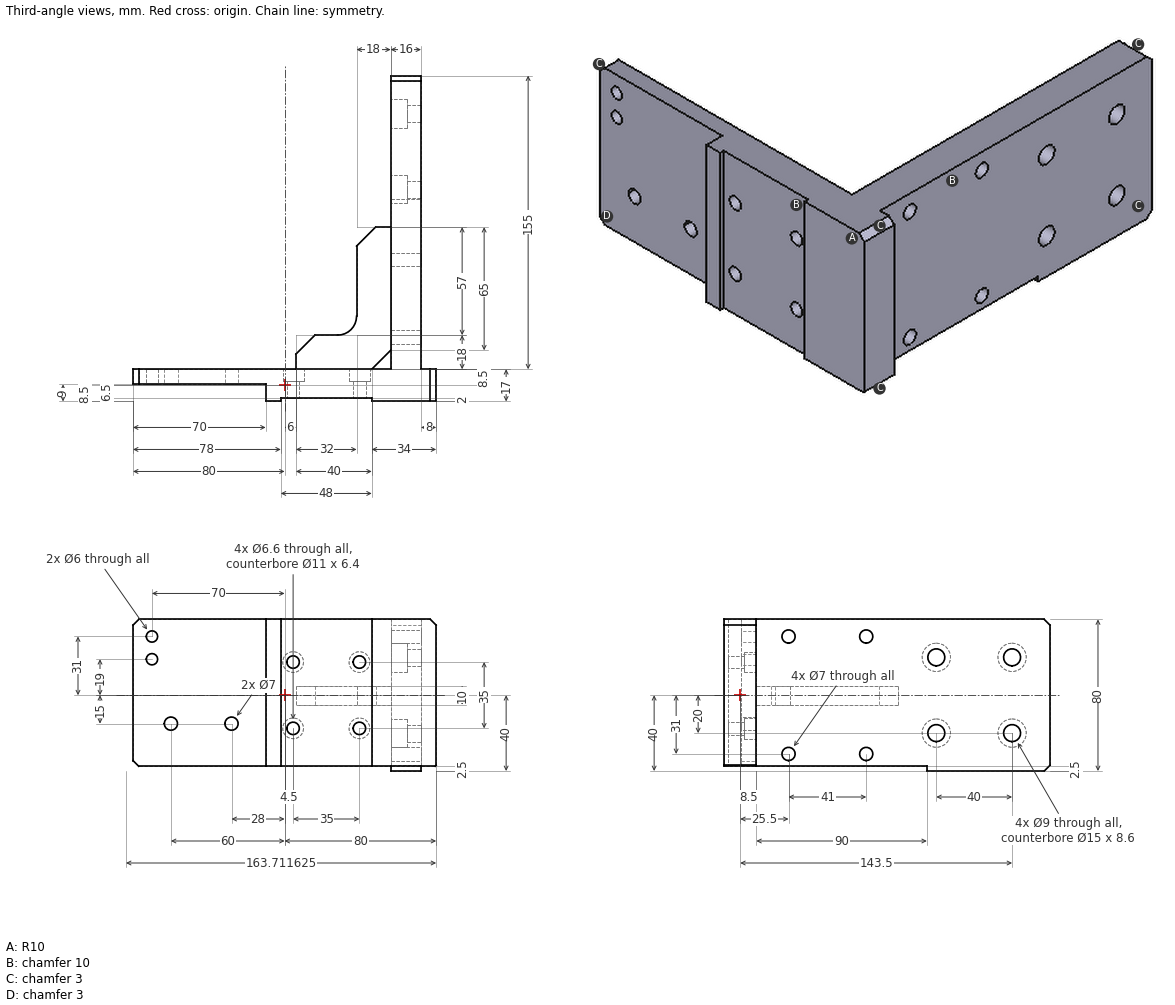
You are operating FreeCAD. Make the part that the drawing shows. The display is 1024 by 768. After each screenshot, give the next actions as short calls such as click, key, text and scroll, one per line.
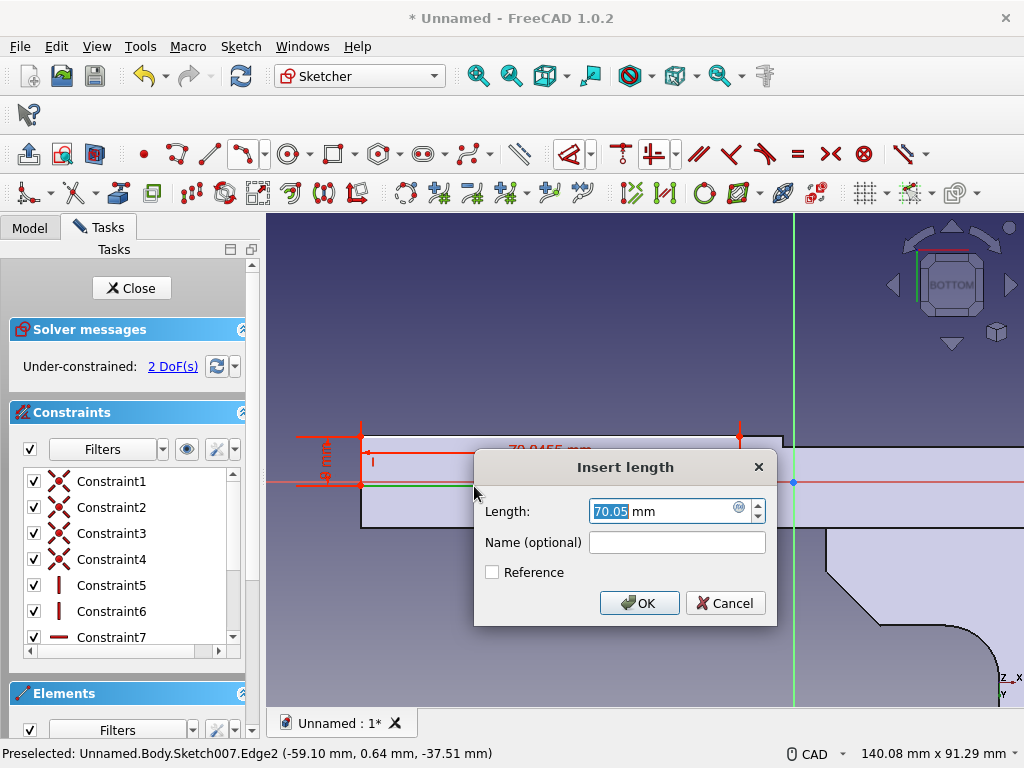
text(70)
key(Return)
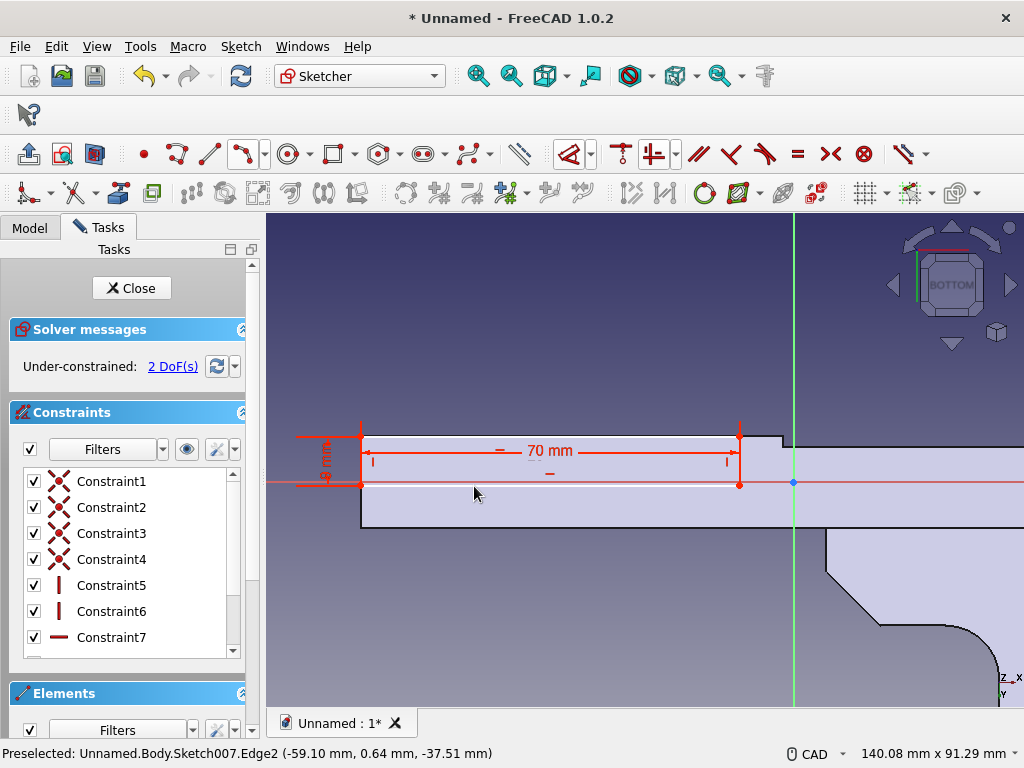
click(361, 437)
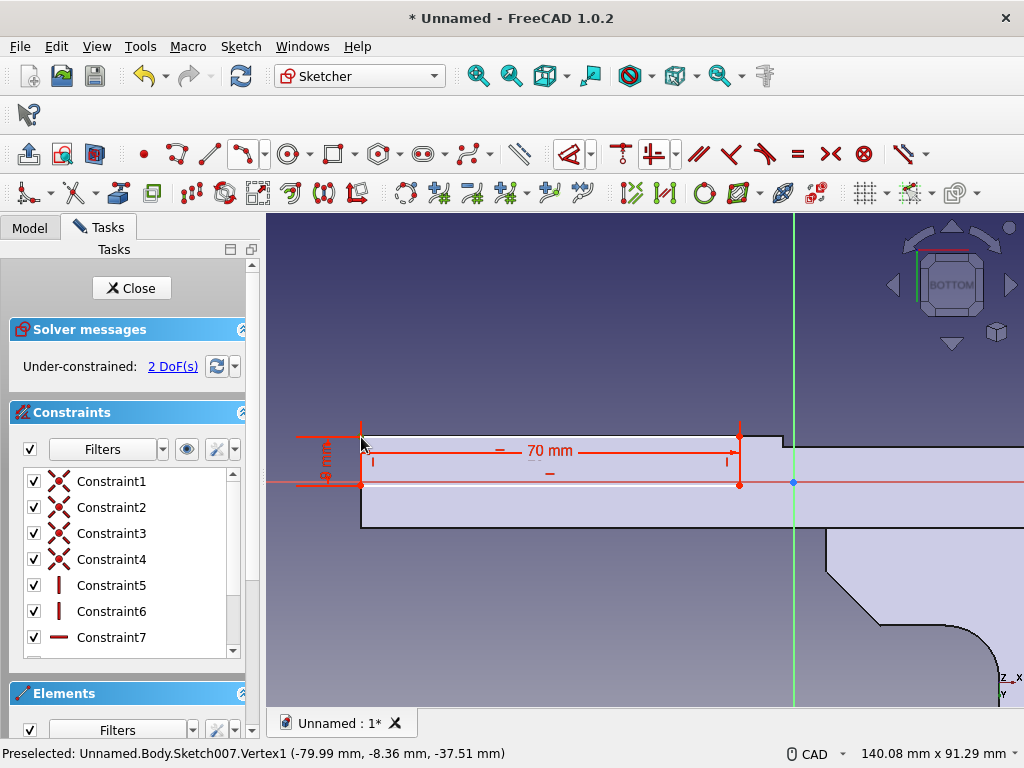
click(590, 154)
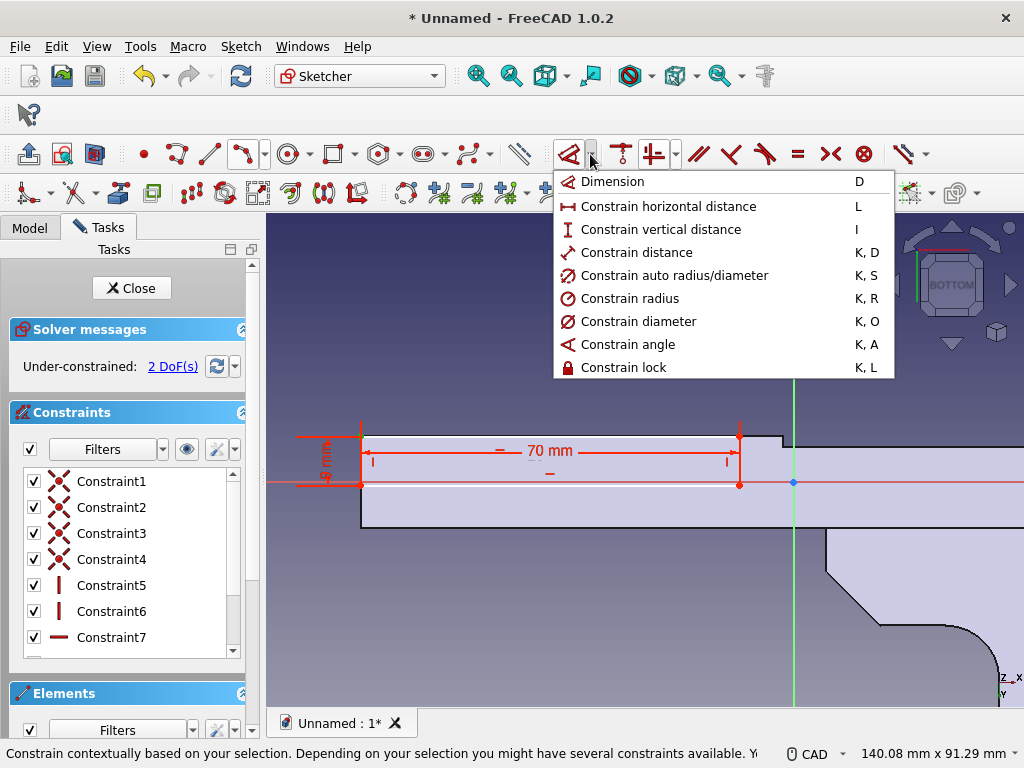
click(724, 206)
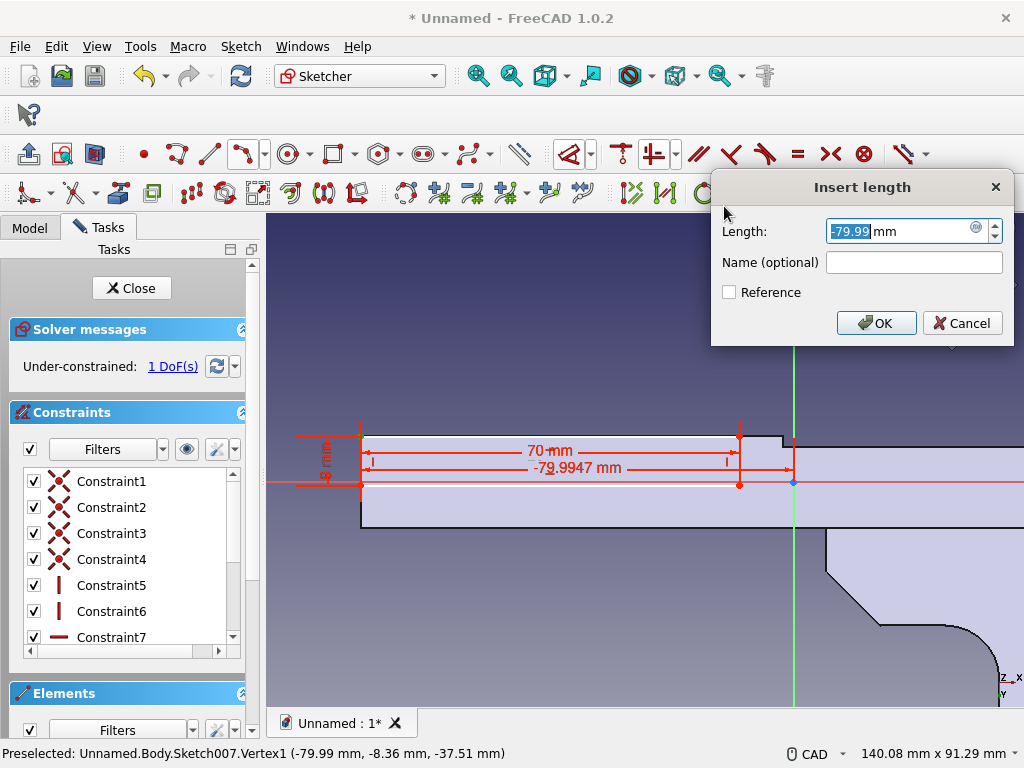
text(-80)
key(Return)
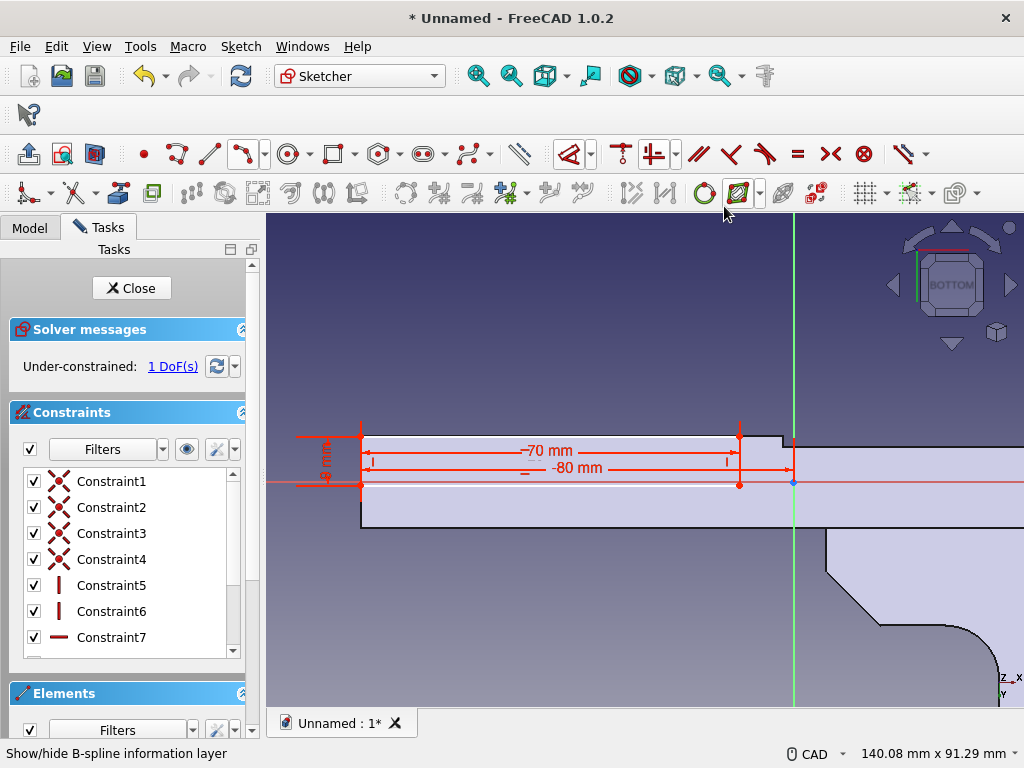
click(361, 437)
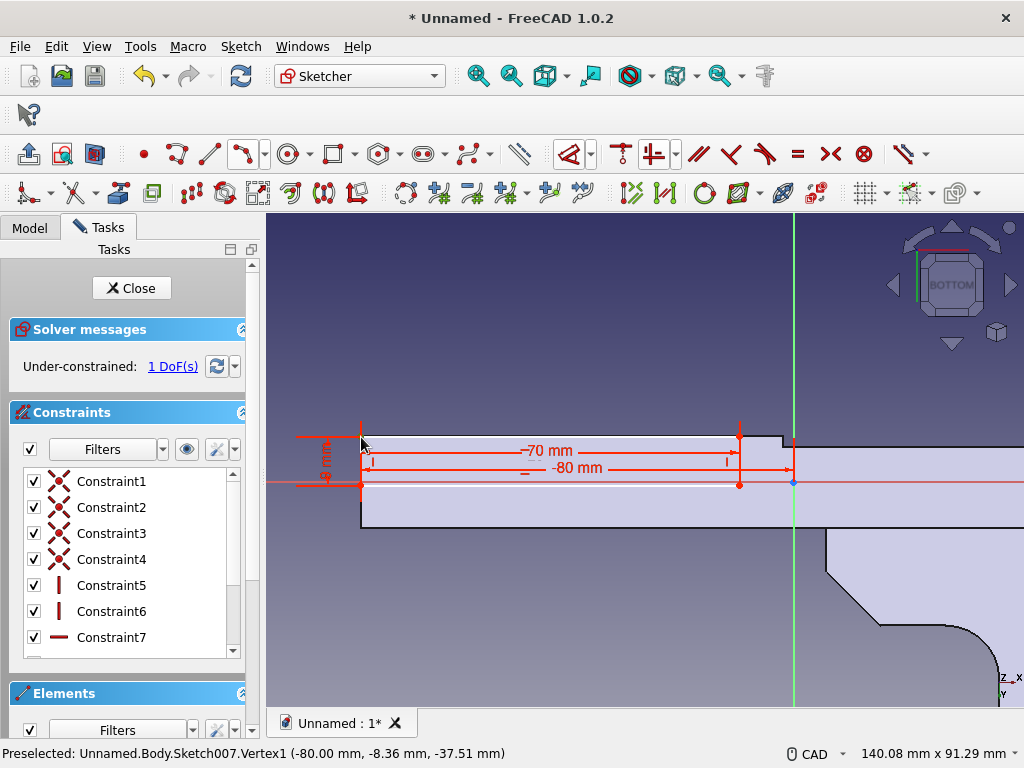
key(i)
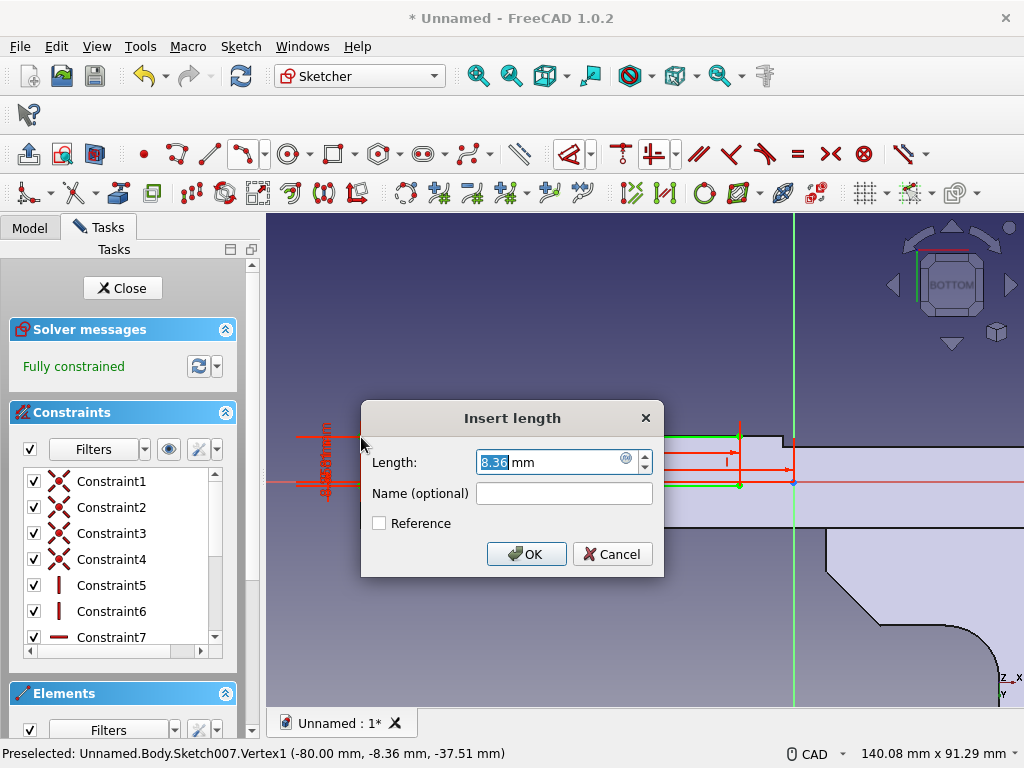
text(8.5)
key(Return)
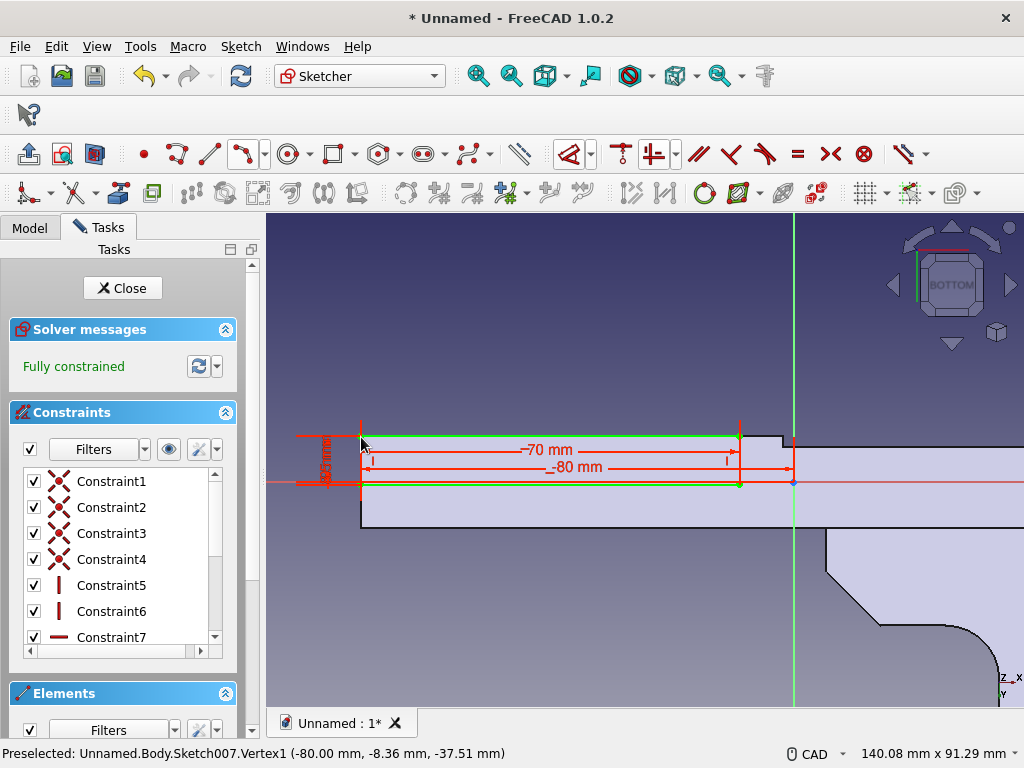
click(123, 288)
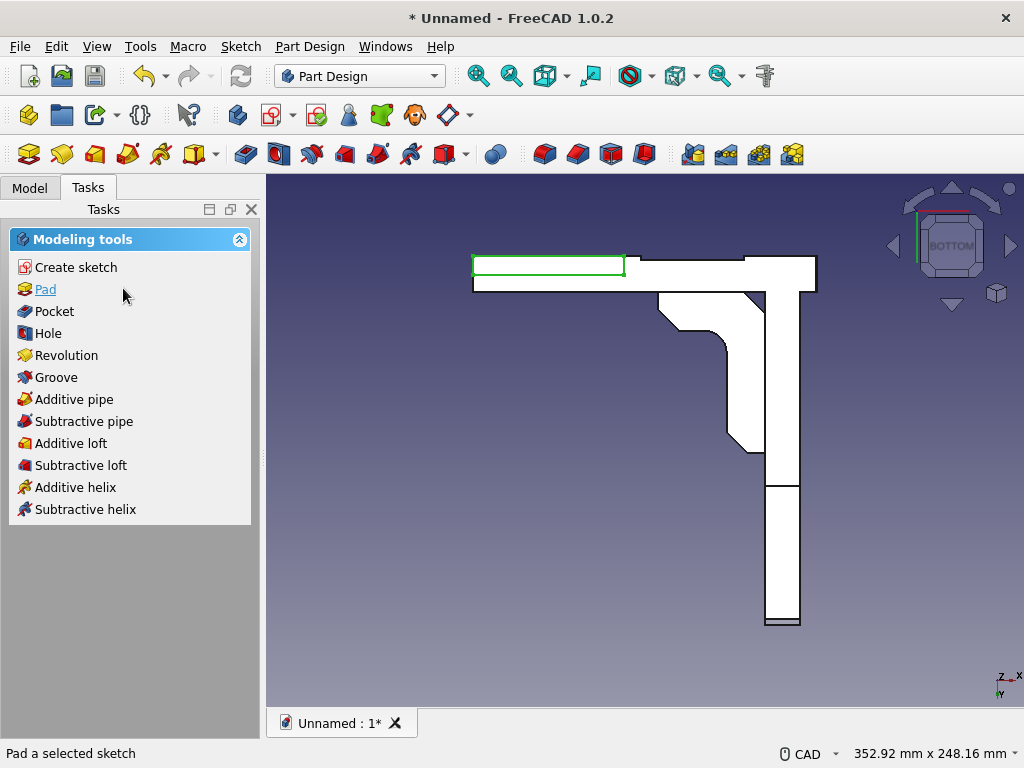
click(246, 154)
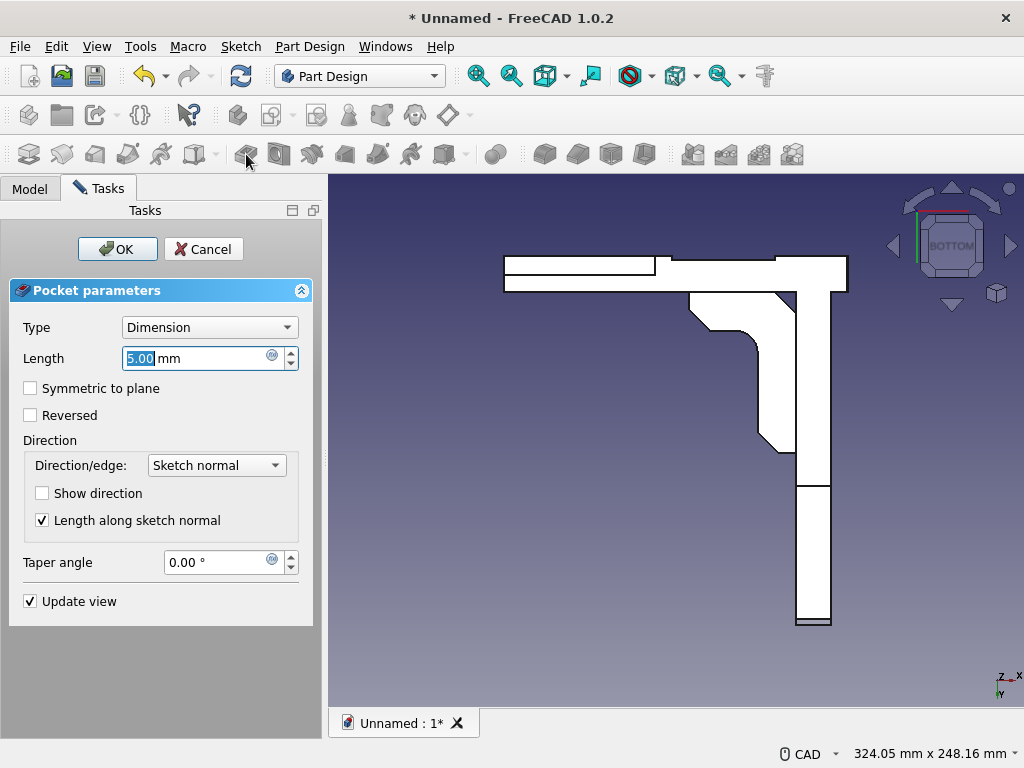
click(210, 328)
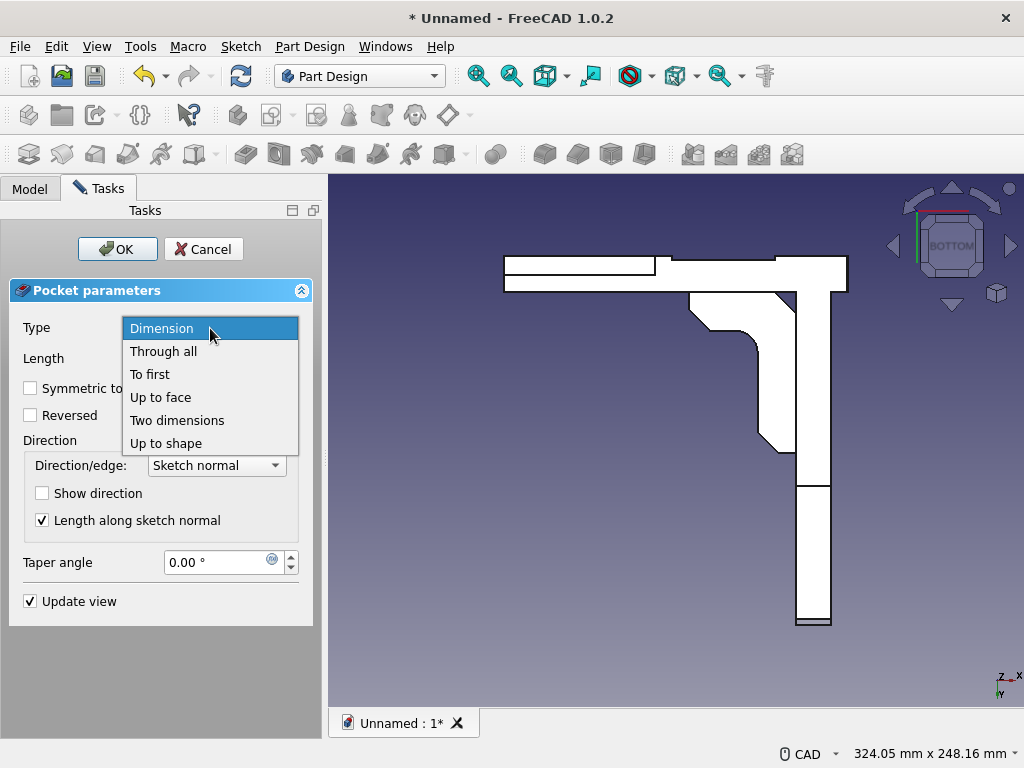
click(208, 352)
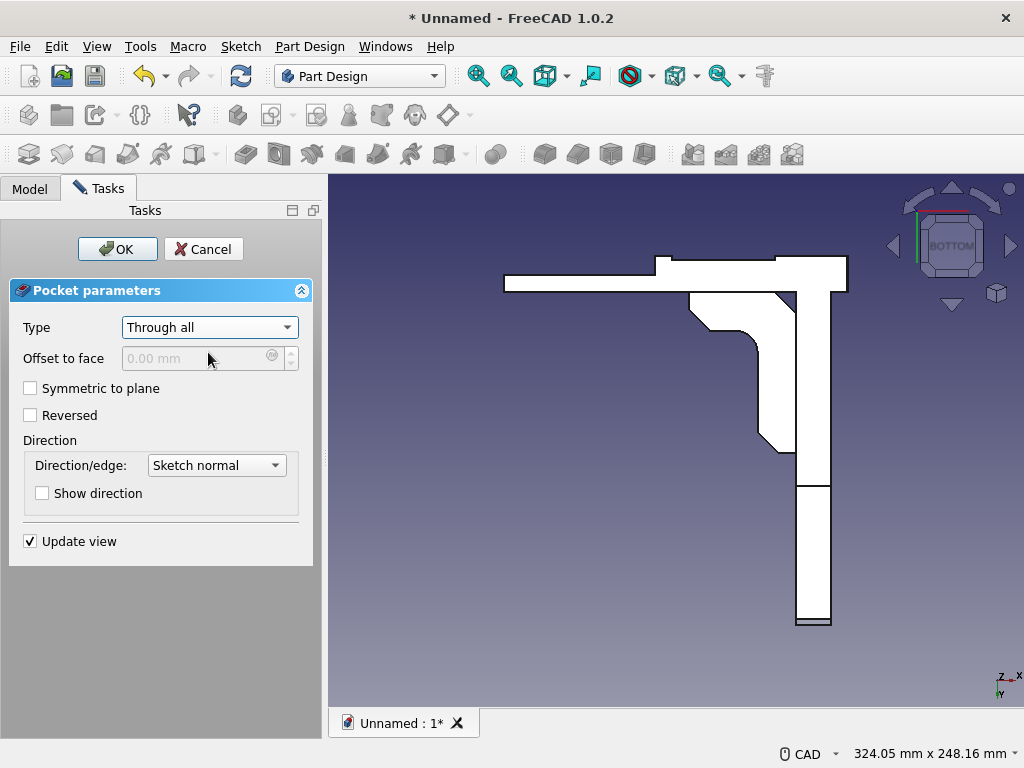
click(118, 249)